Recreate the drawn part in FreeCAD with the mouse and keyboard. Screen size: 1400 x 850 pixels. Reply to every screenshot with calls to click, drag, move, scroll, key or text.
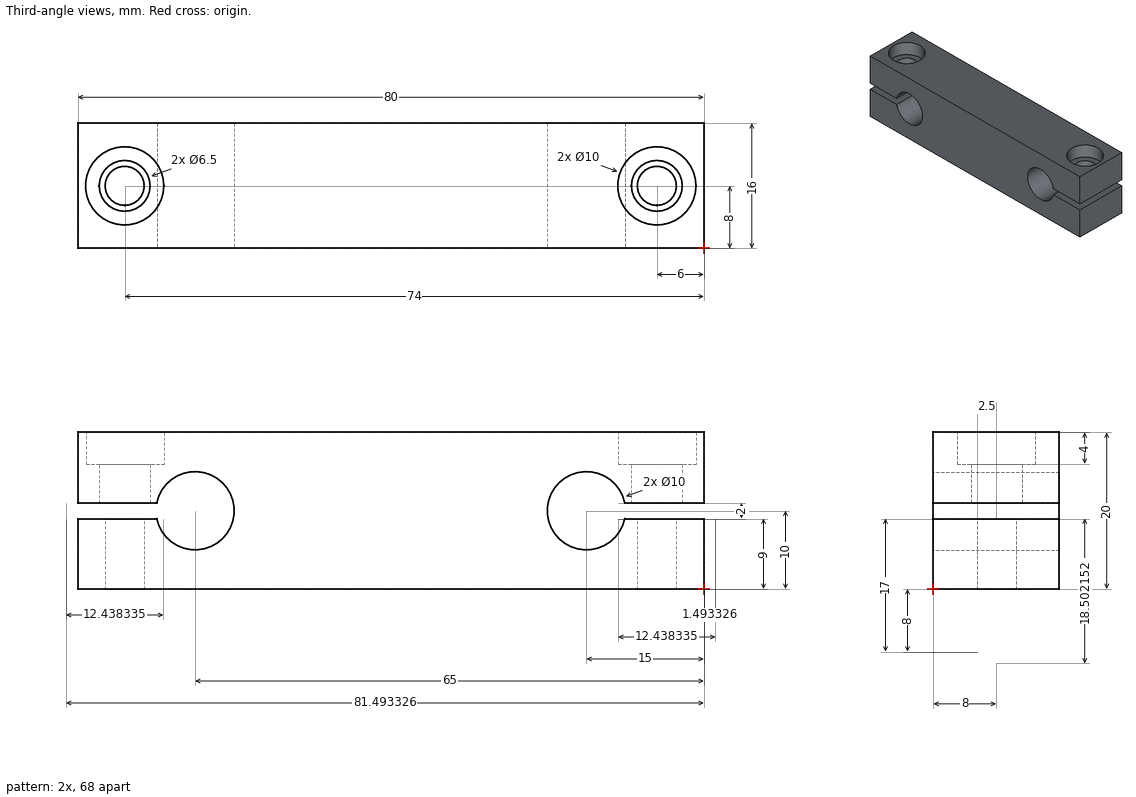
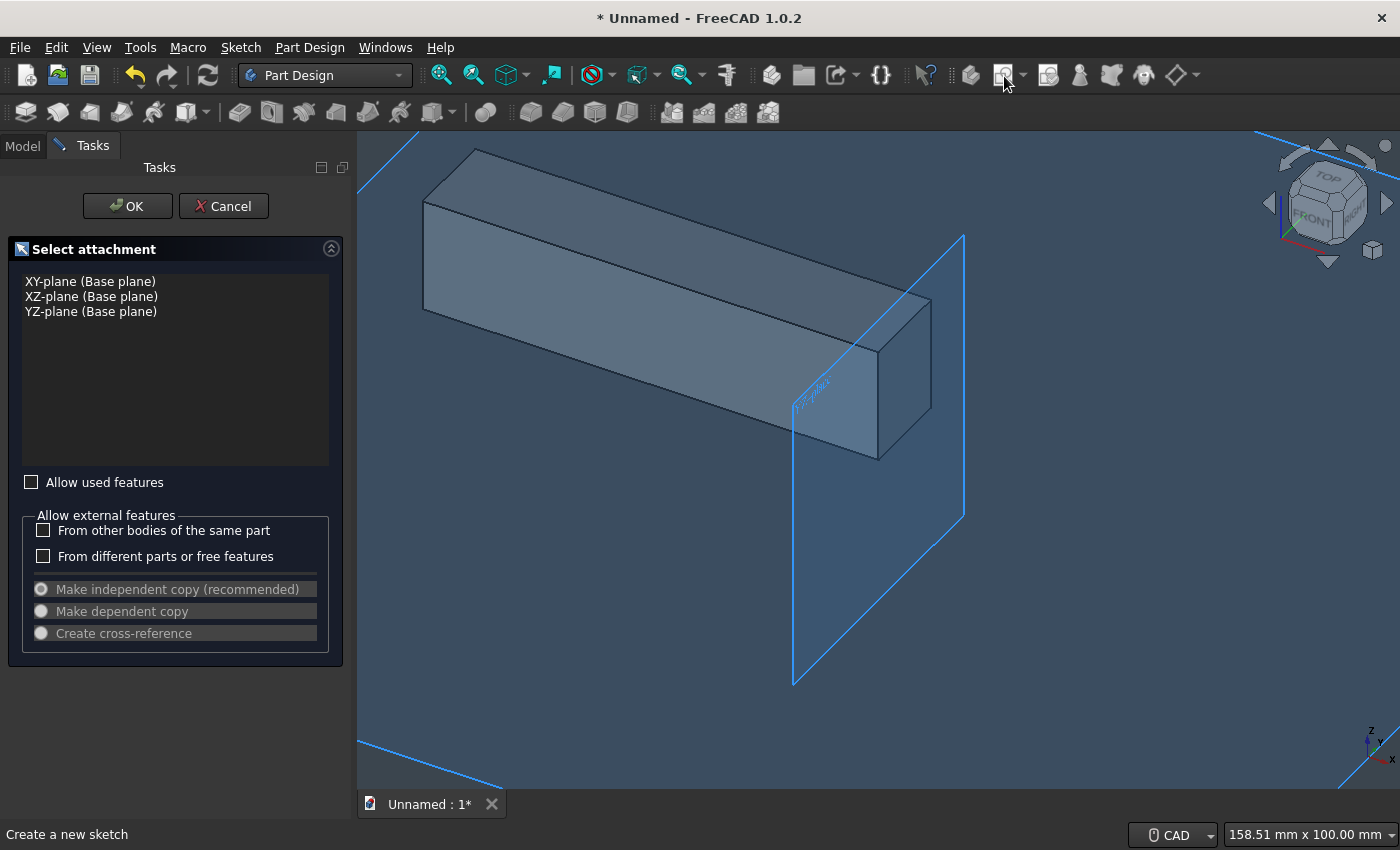
click(82, 296)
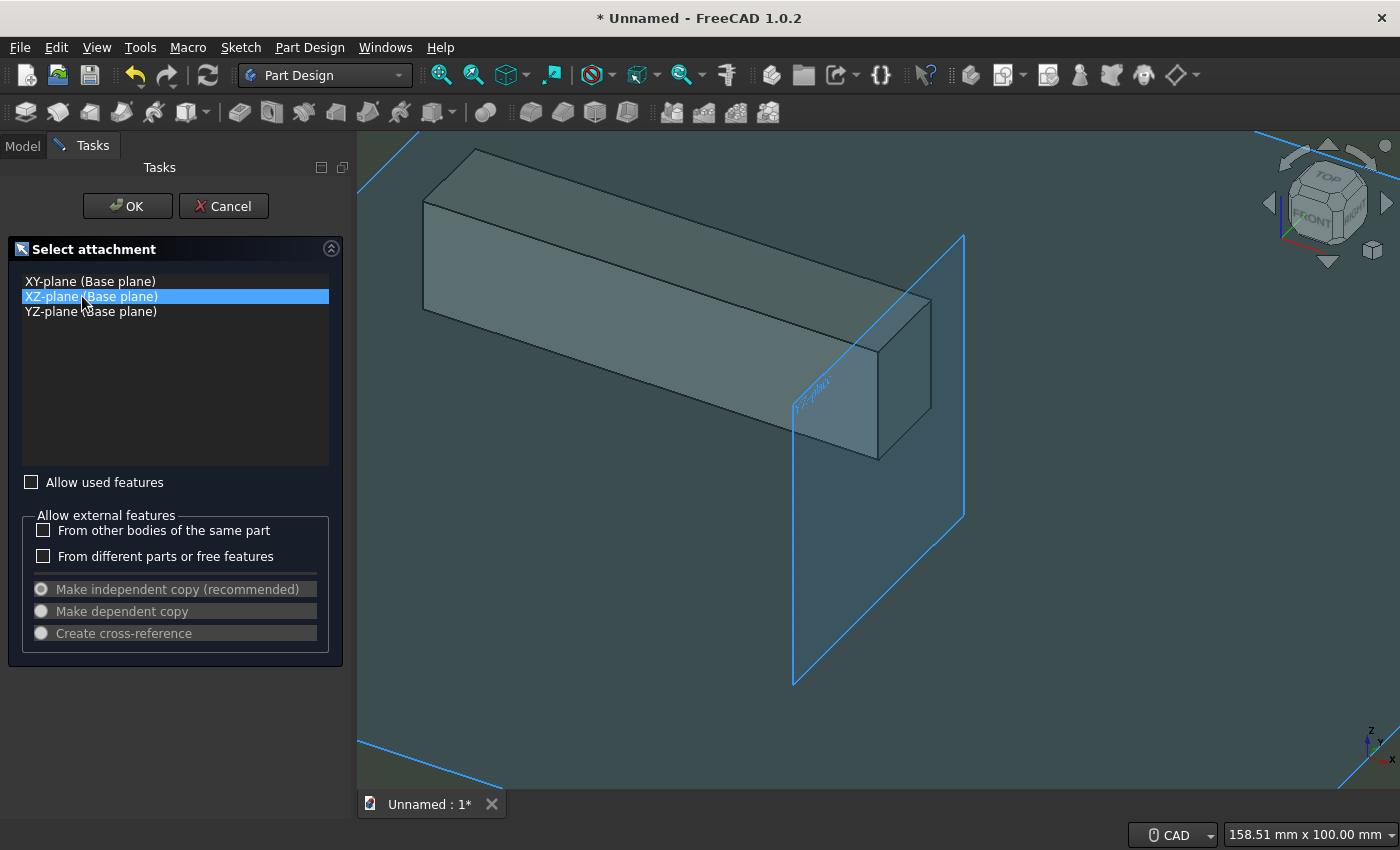
click(128, 206)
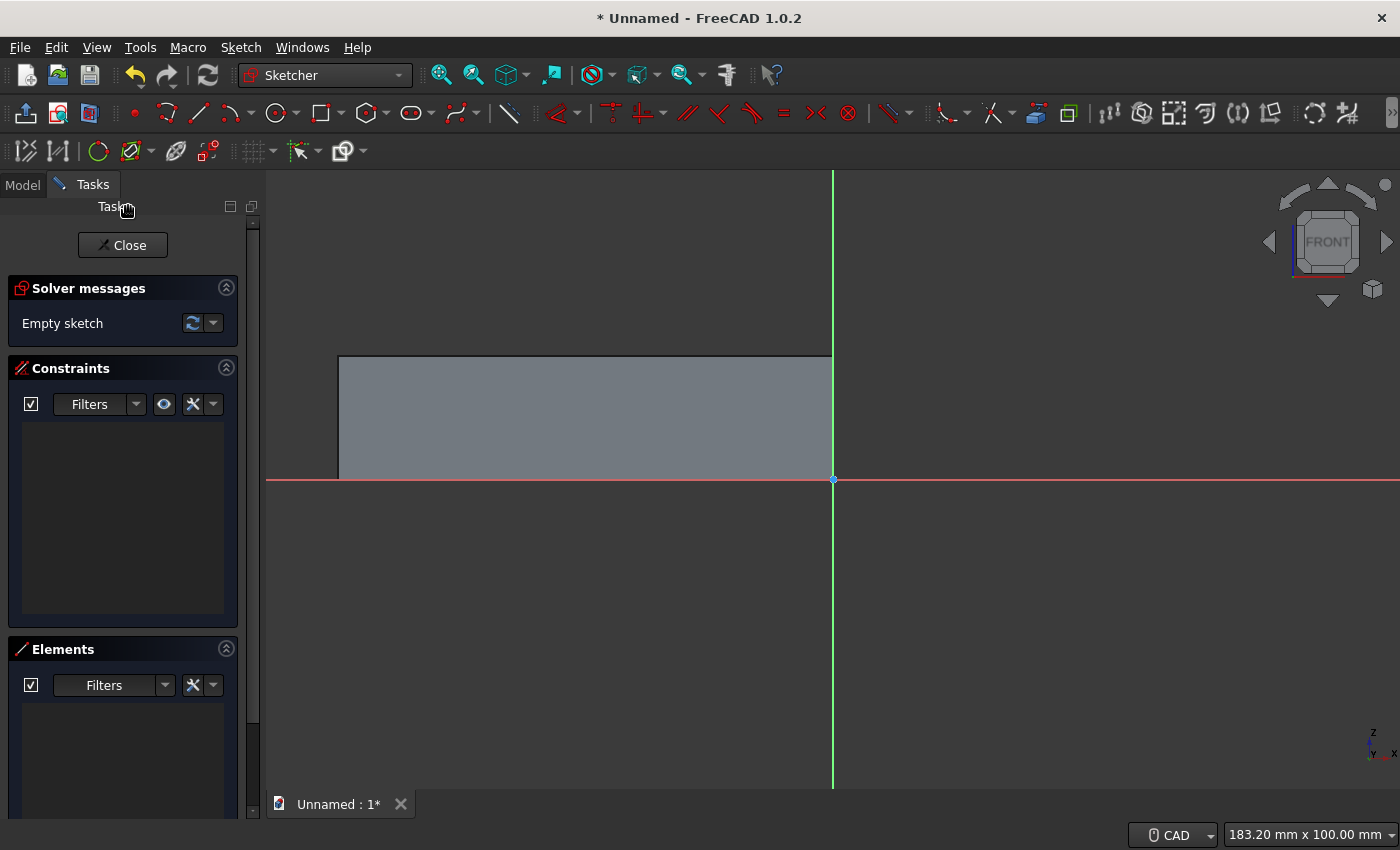
scroll(315, 339, up, 2)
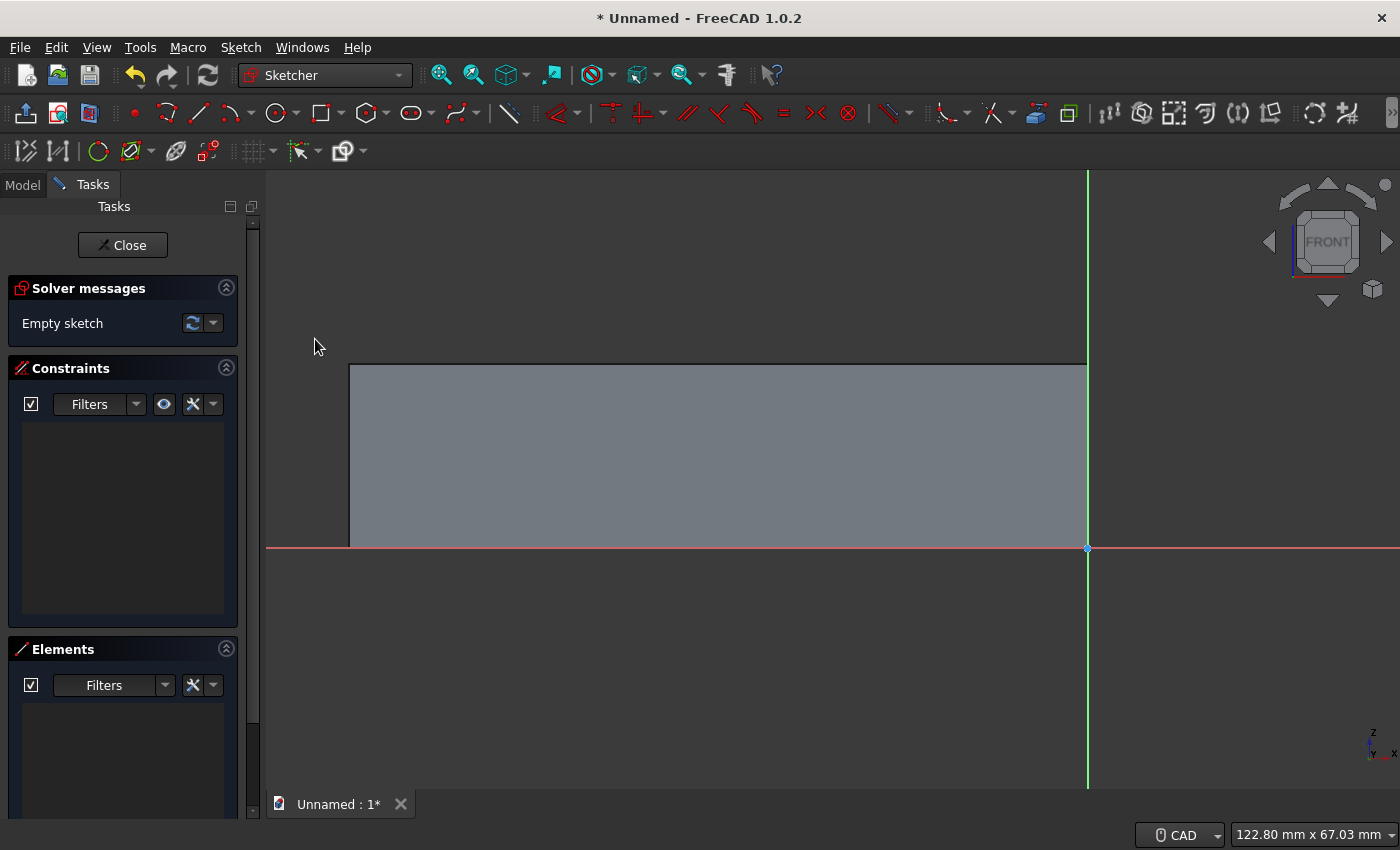
click(276, 114)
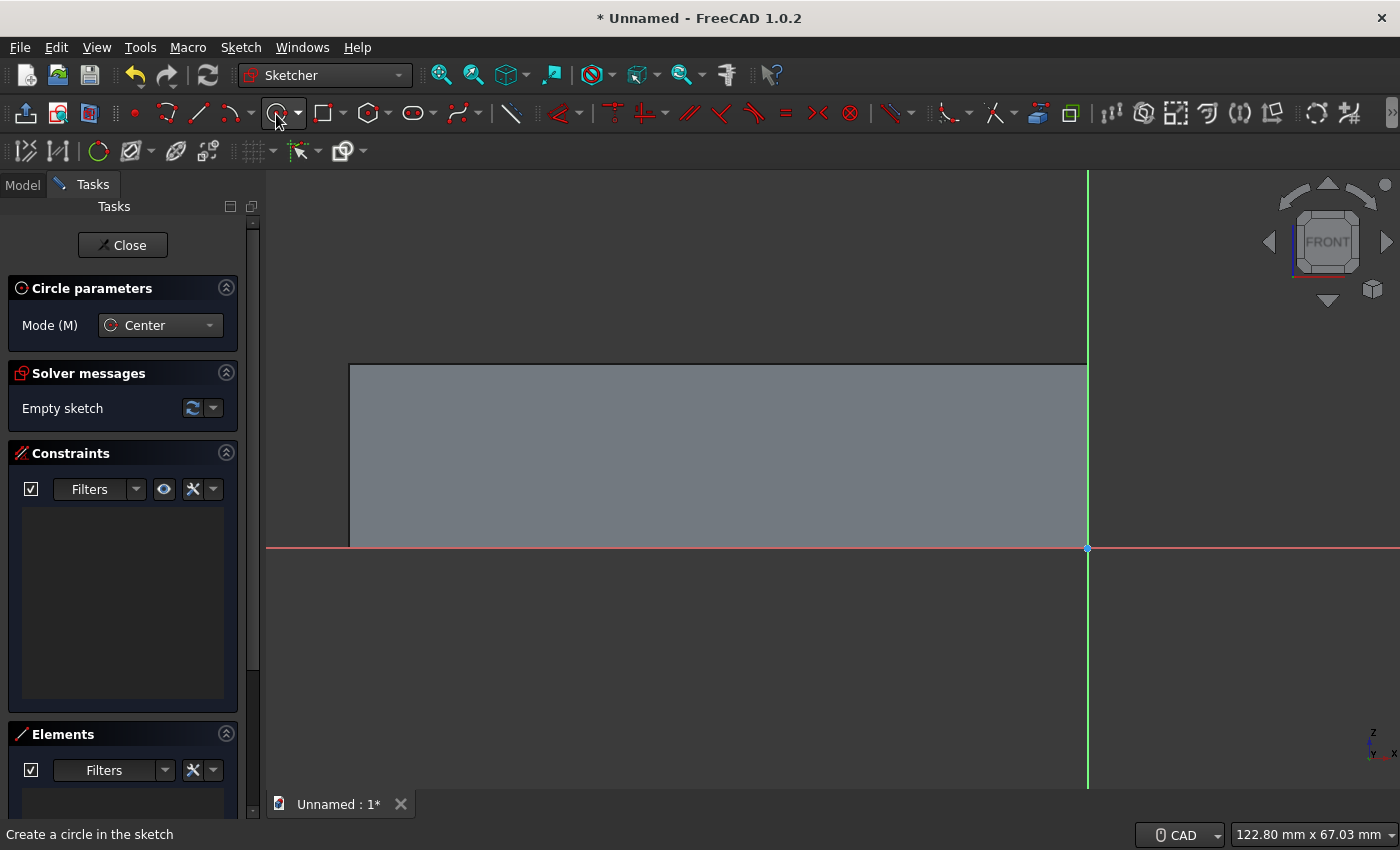
click(949, 456)
click(982, 423)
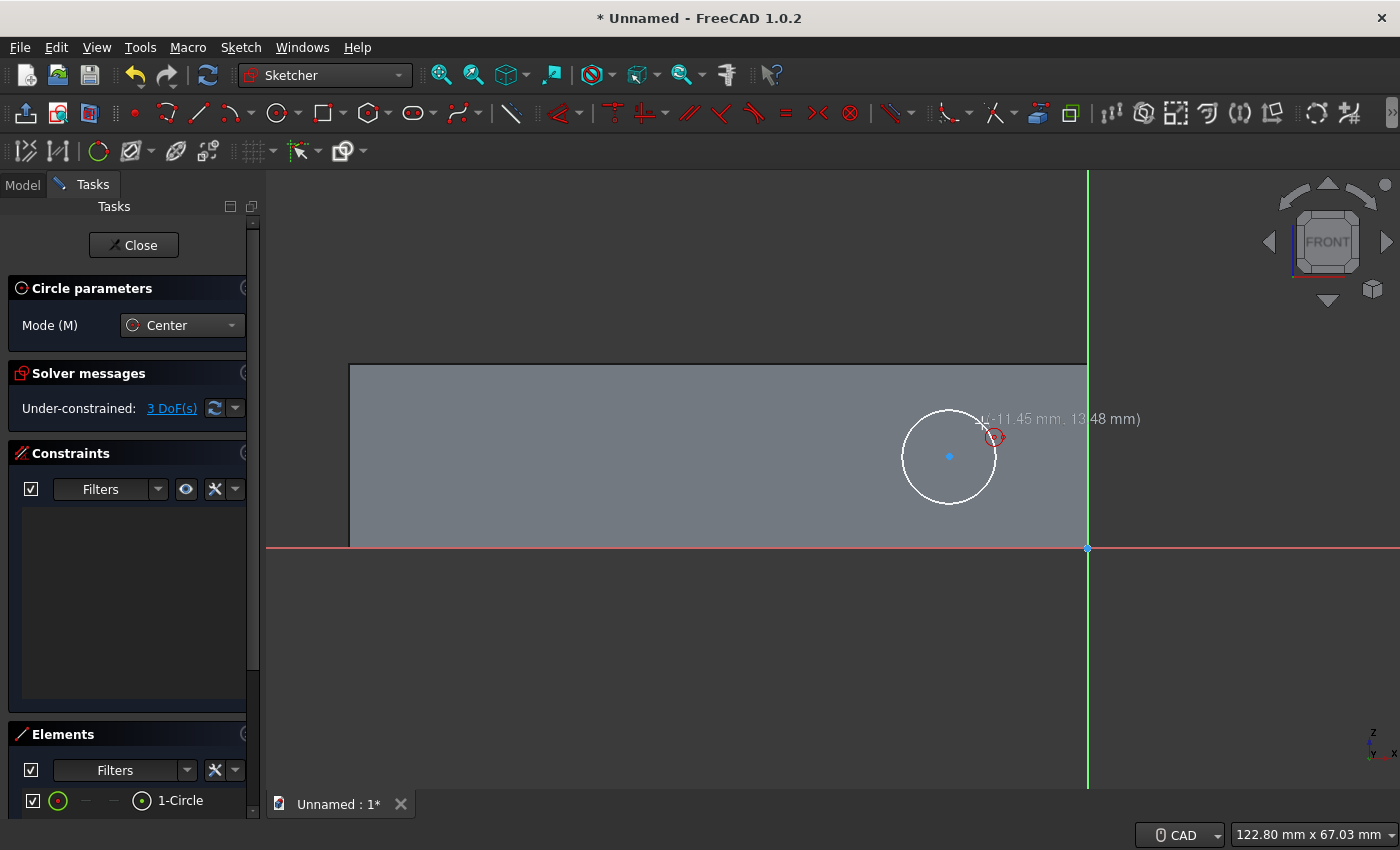
click(488, 456)
click(520, 423)
key(Escape)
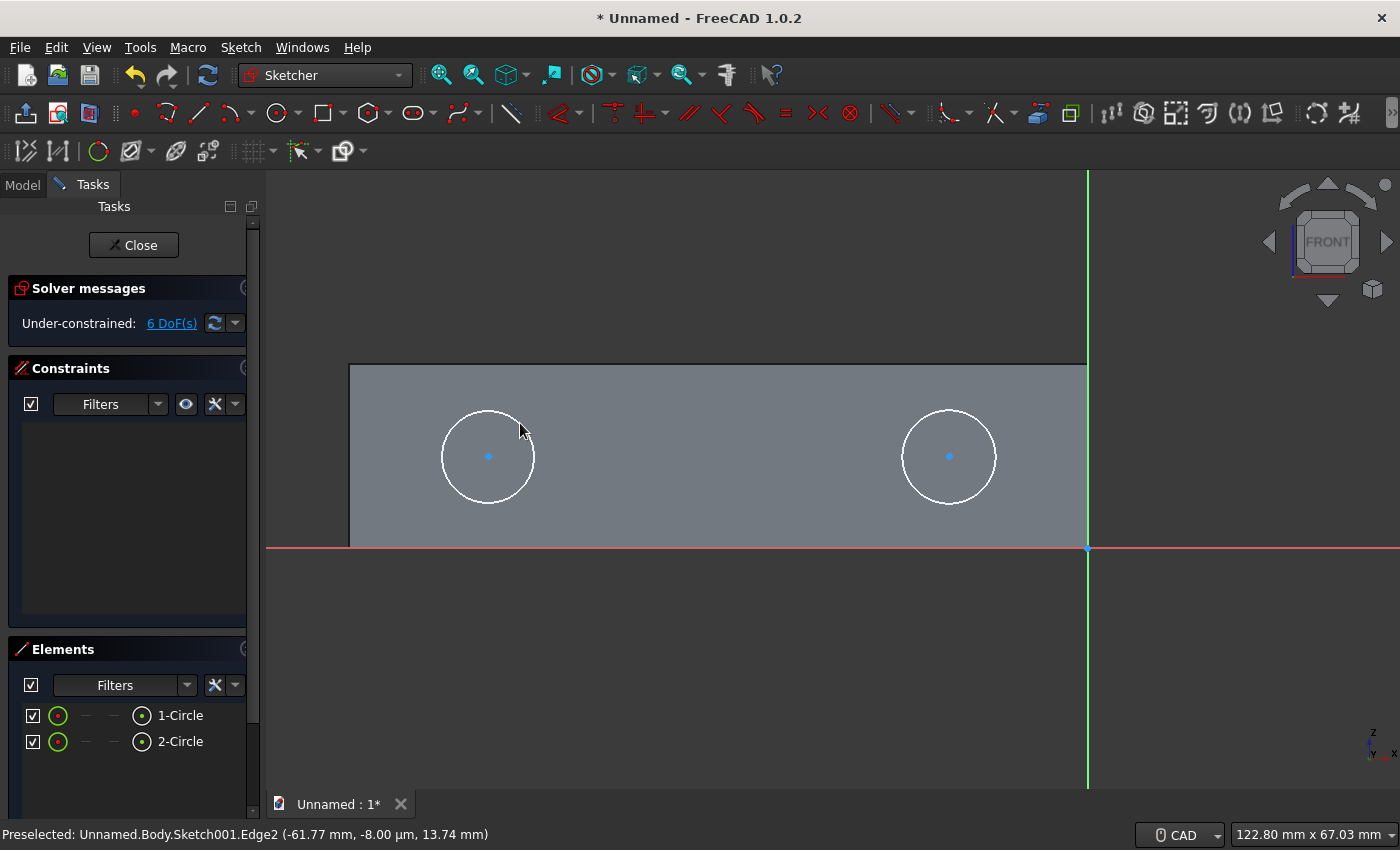
click(982, 424)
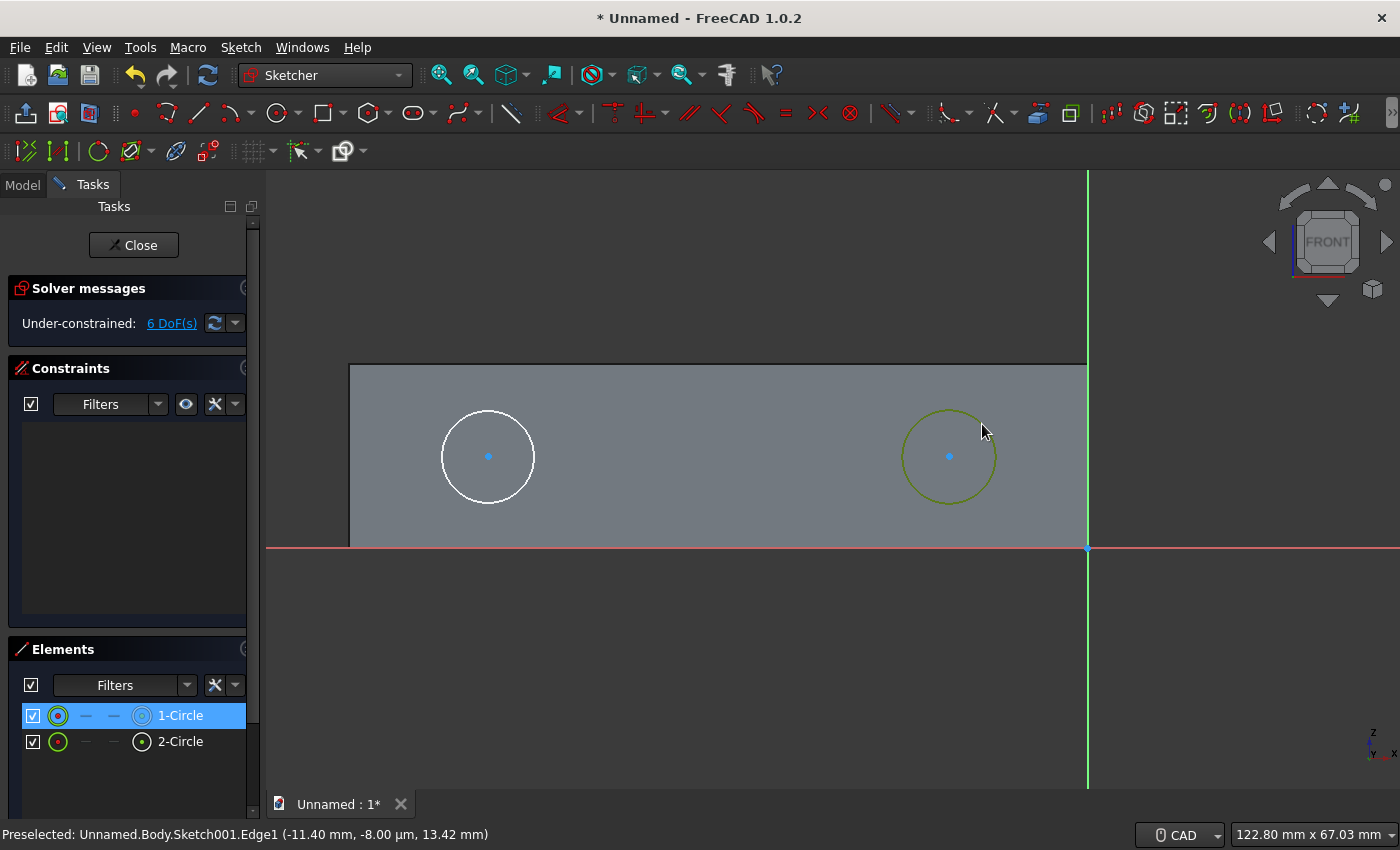
click(520, 424)